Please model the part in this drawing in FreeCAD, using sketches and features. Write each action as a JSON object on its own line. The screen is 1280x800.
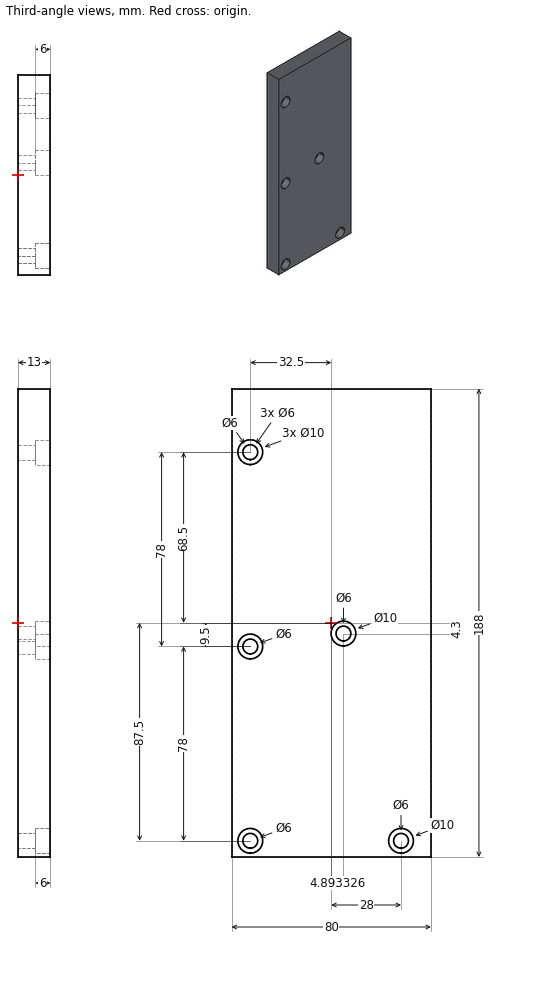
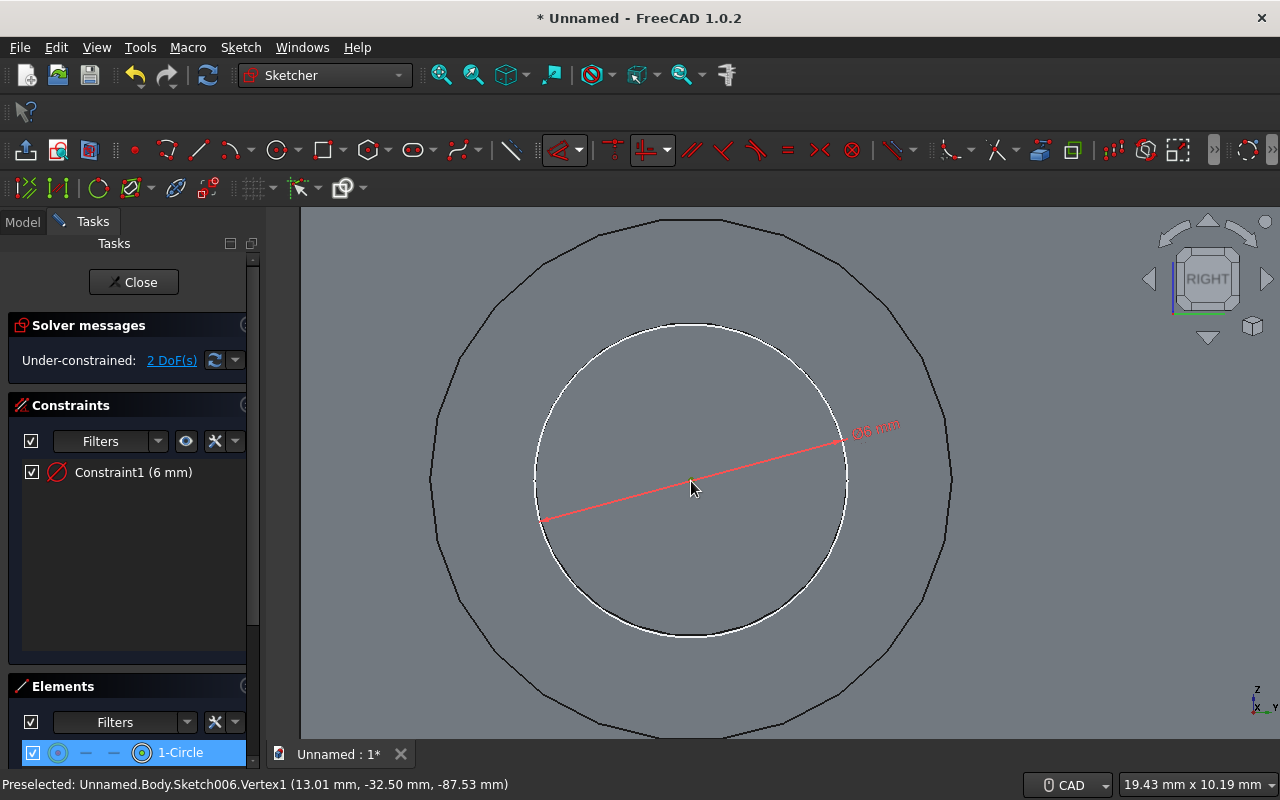
{"action": "left_click", "coordinate": [582, 150]}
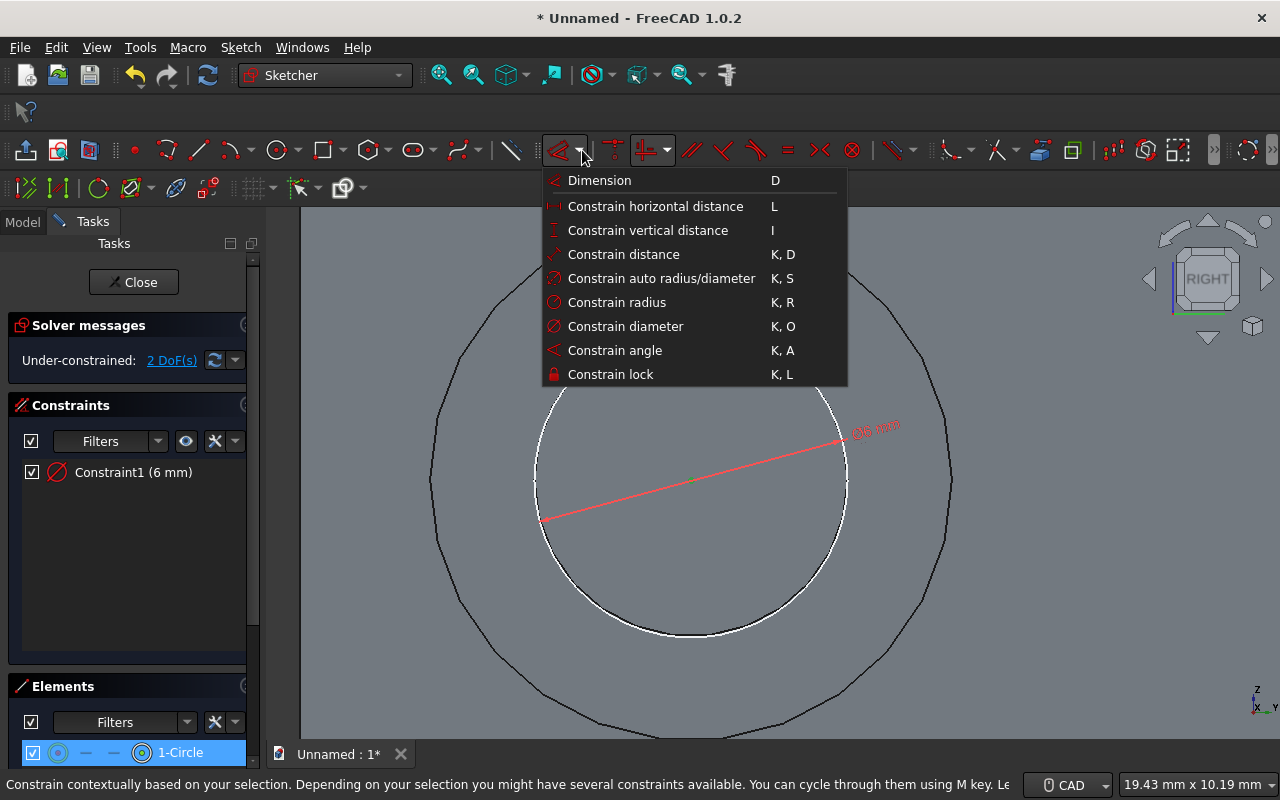
{"action": "left_click", "coordinate": [695, 206]}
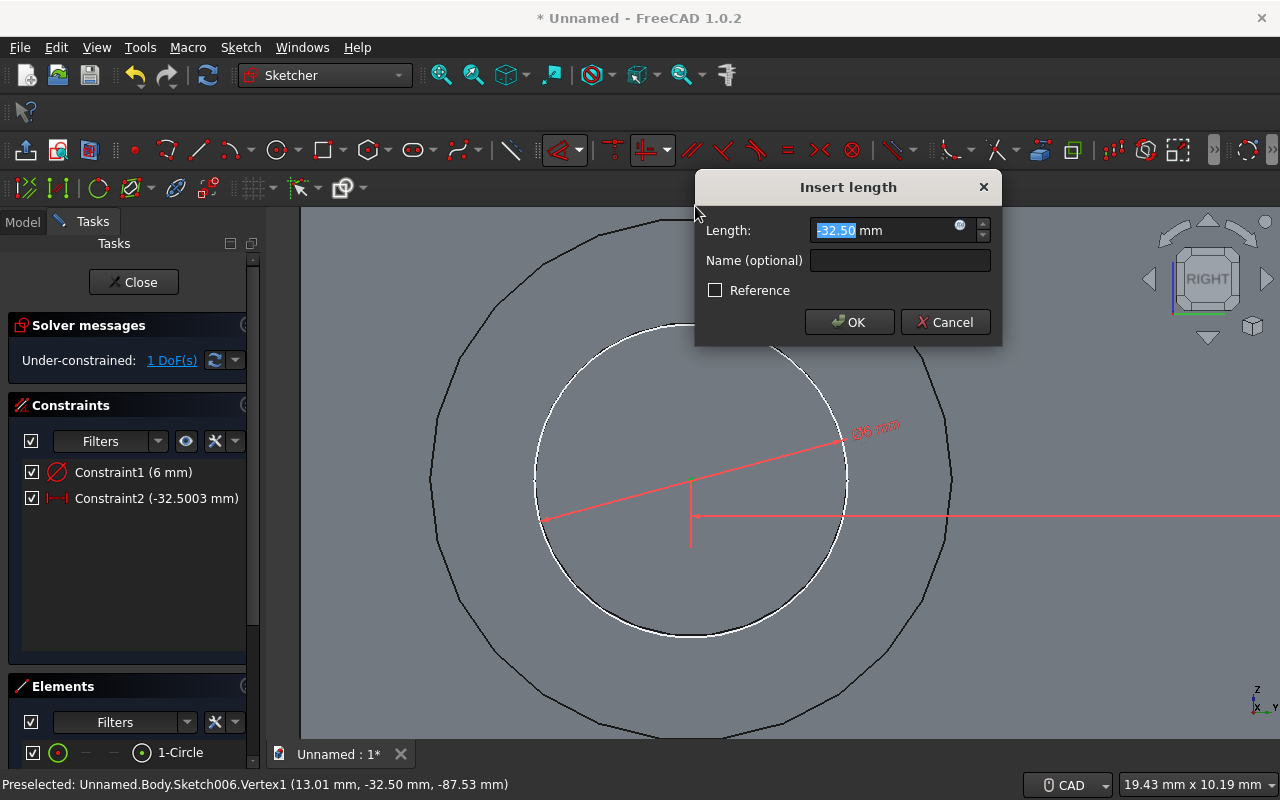
{"action": "type", "text": "-32.5"}
{"action": "key", "text": "Return"}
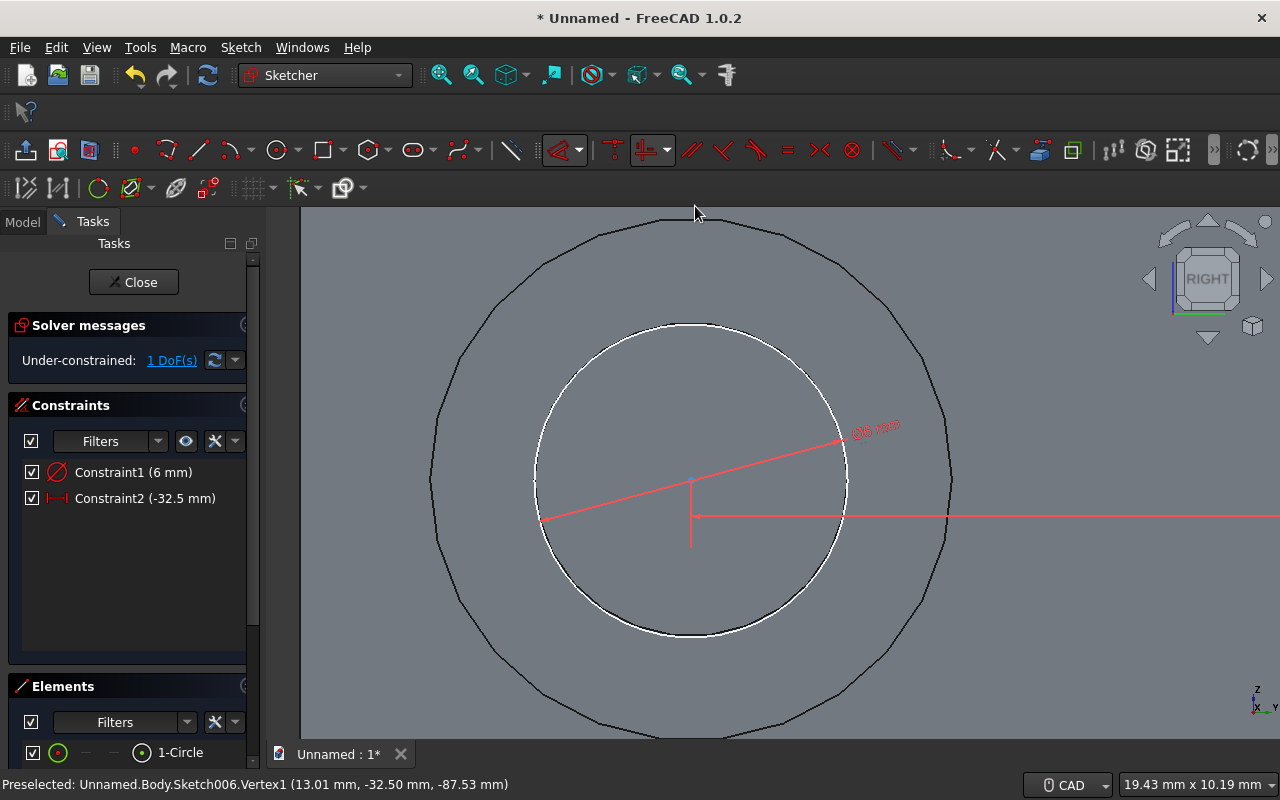
{"action": "left_click", "coordinate": [691, 481]}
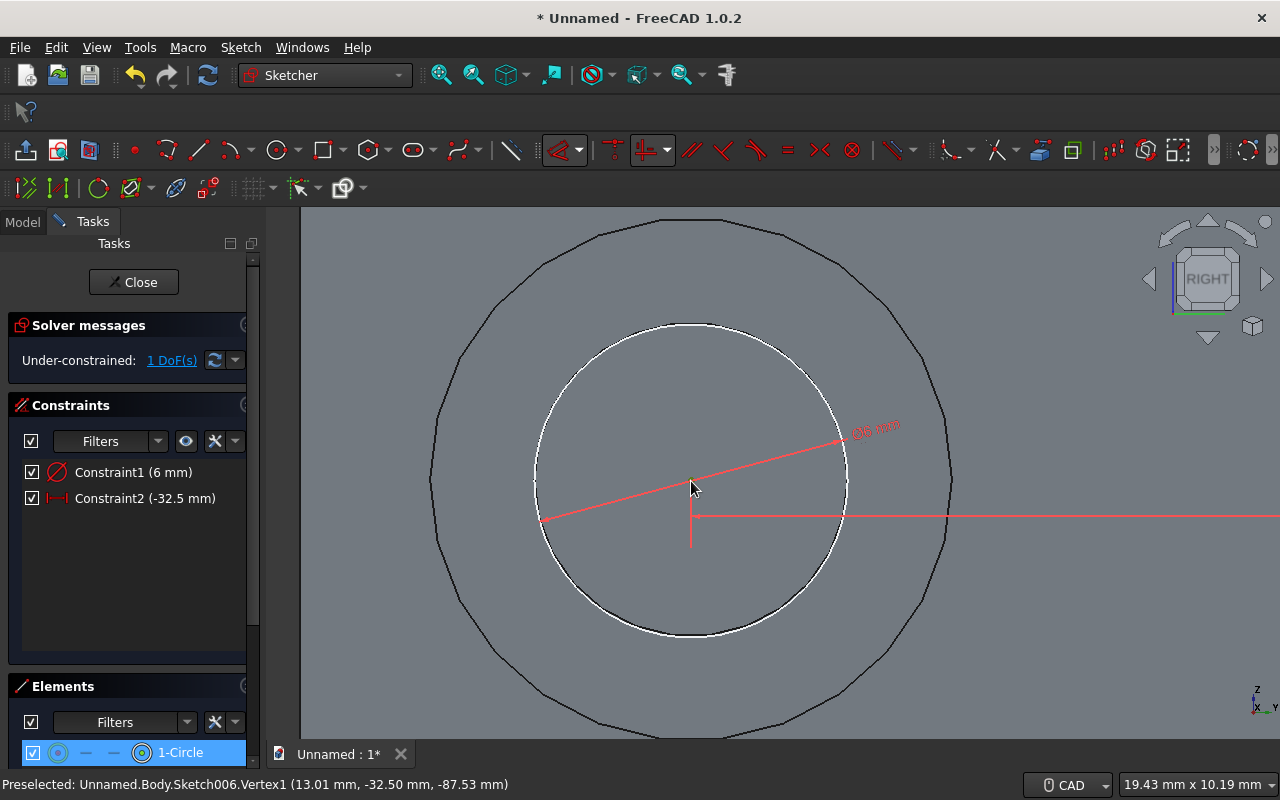
{"action": "left_click", "coordinate": [582, 150]}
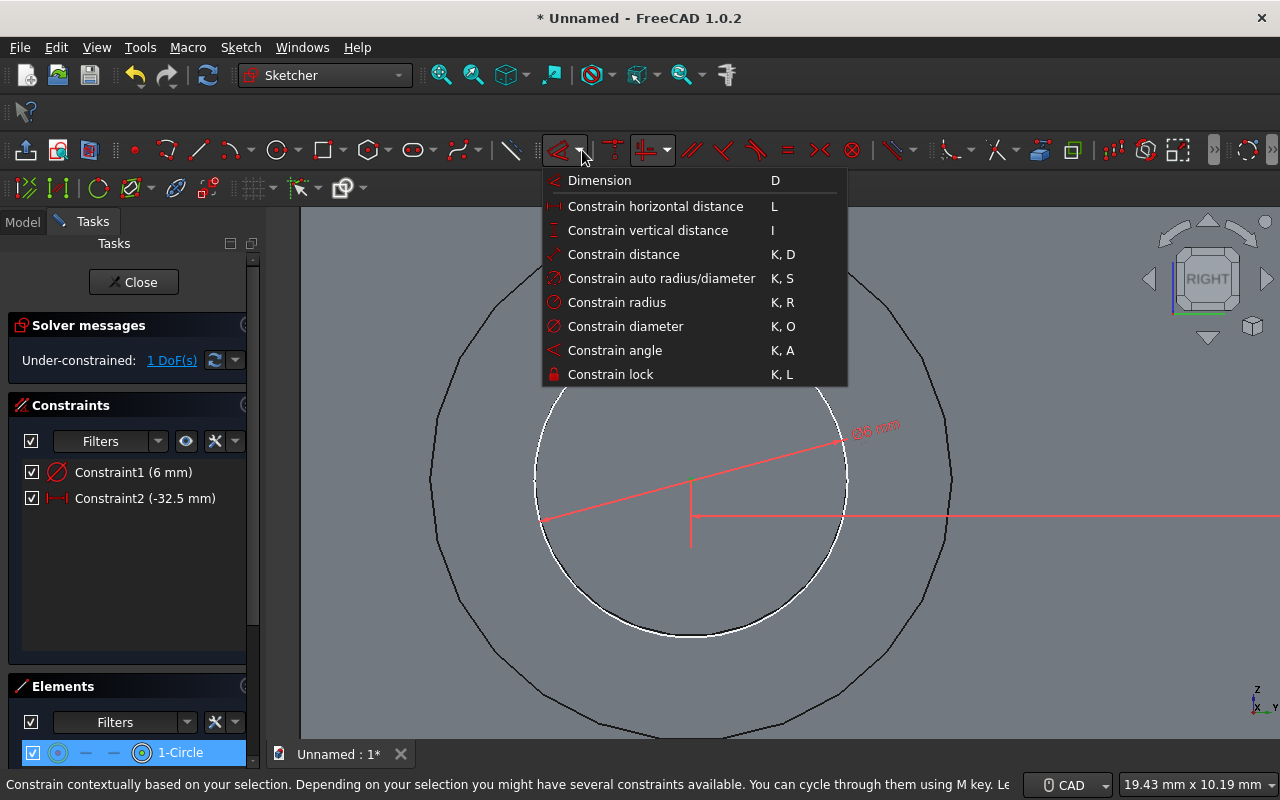
{"action": "left_click", "coordinate": [695, 230]}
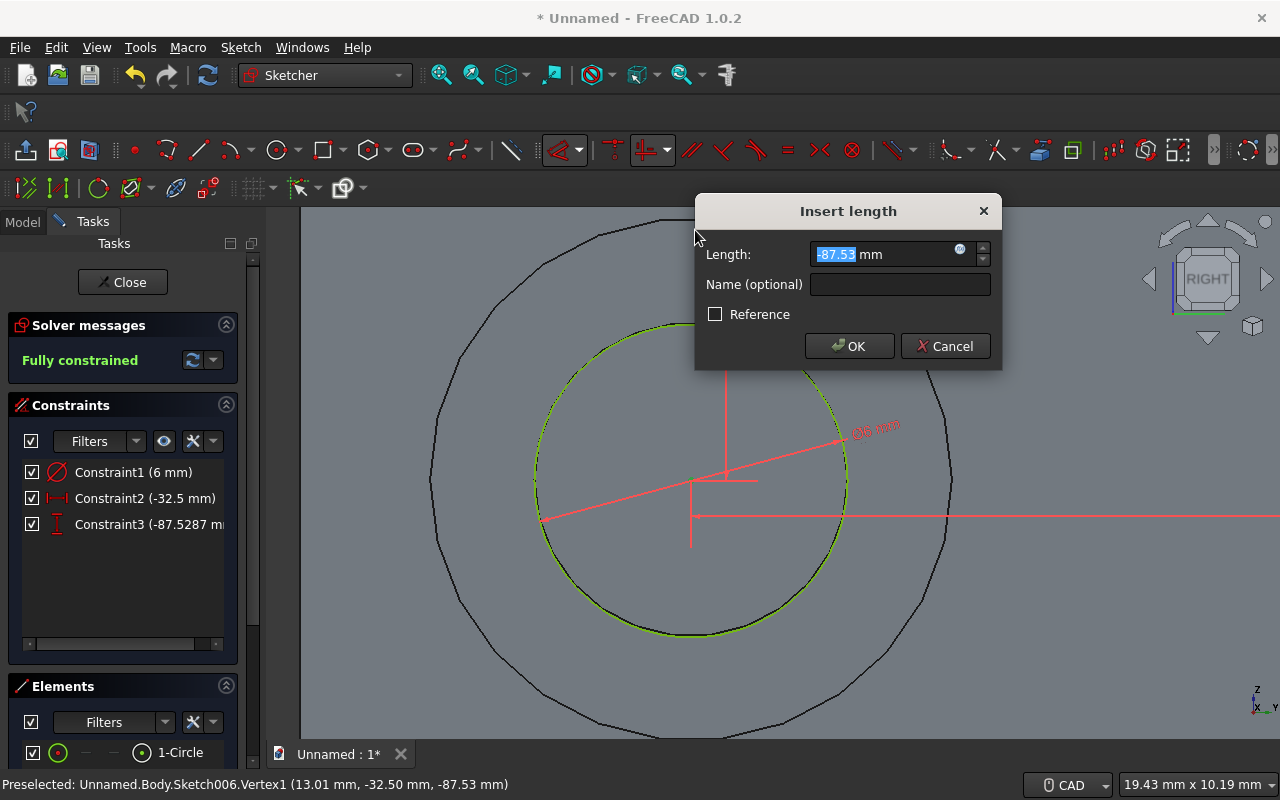
{"action": "type", "text": "-87.5"}
{"action": "key", "text": "Return"}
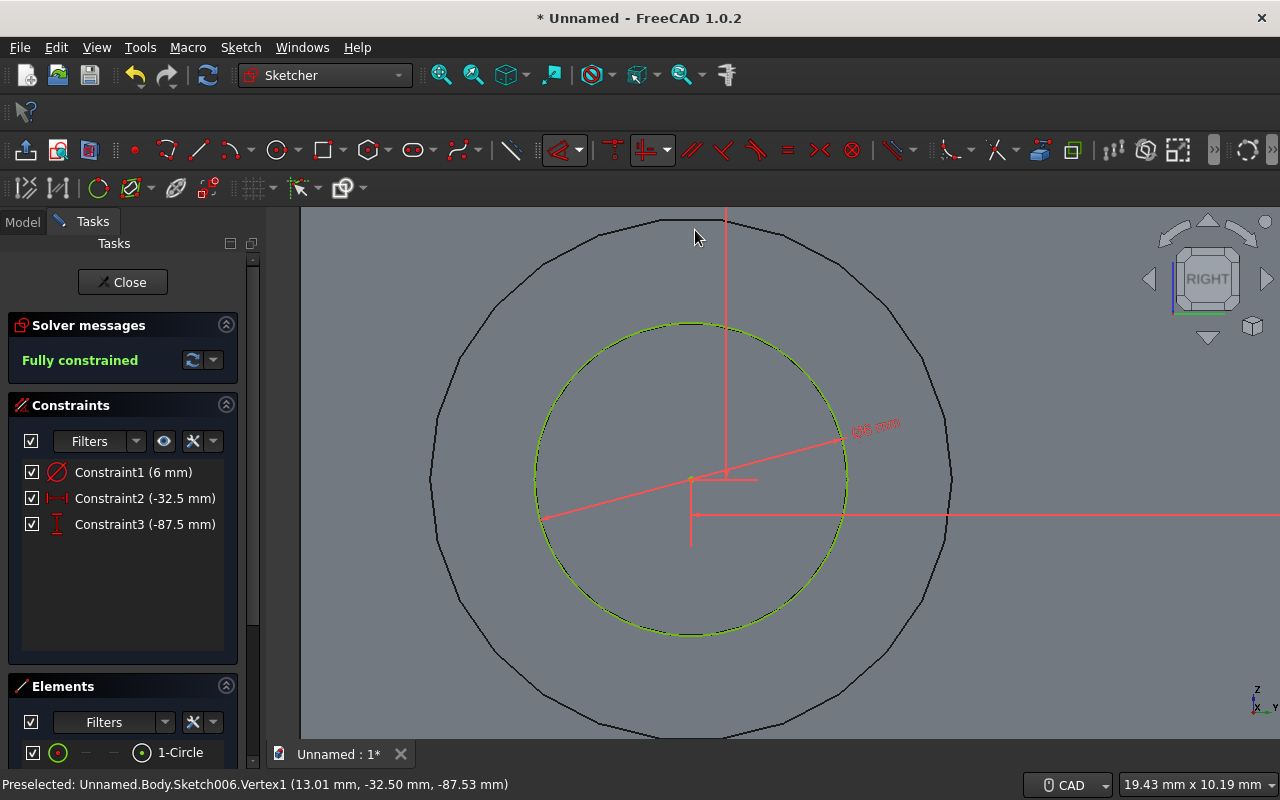
{"action": "left_click", "coordinate": [123, 282]}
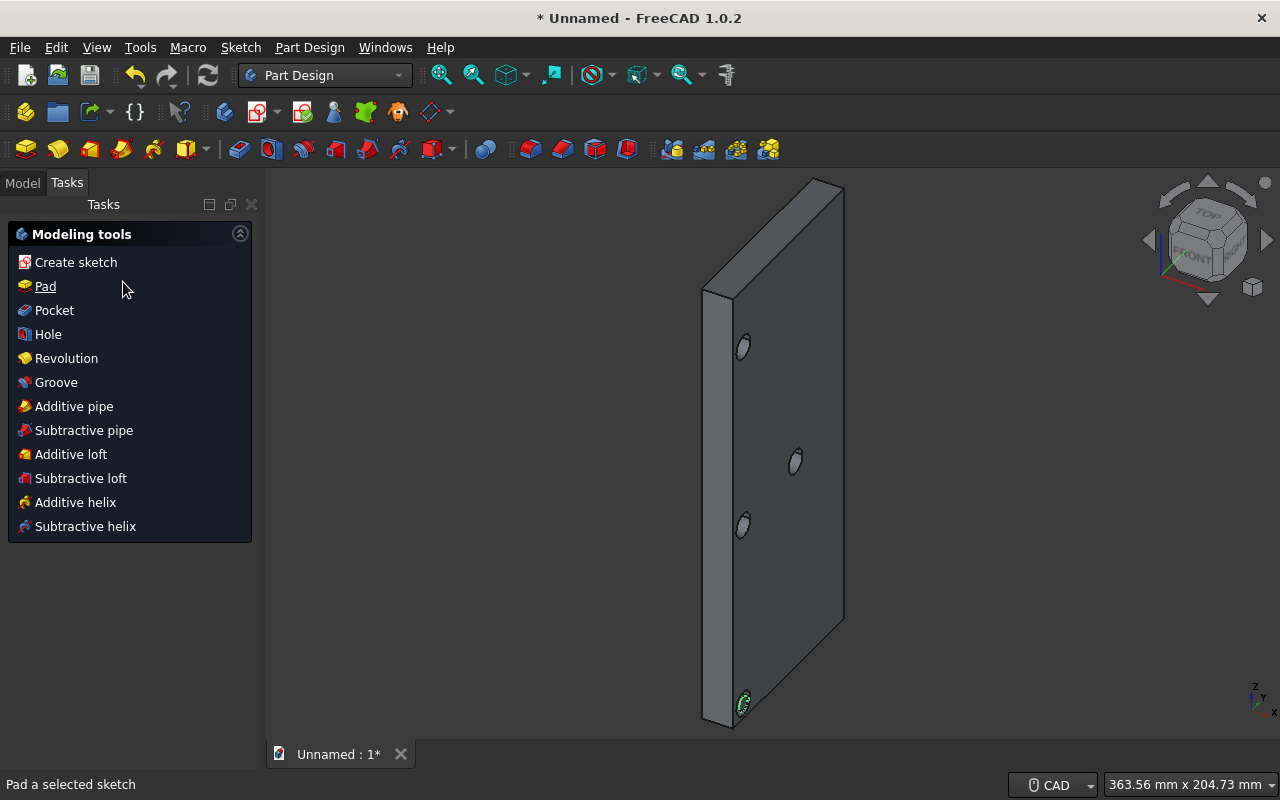
{"action": "left_click", "coordinate": [240, 150]}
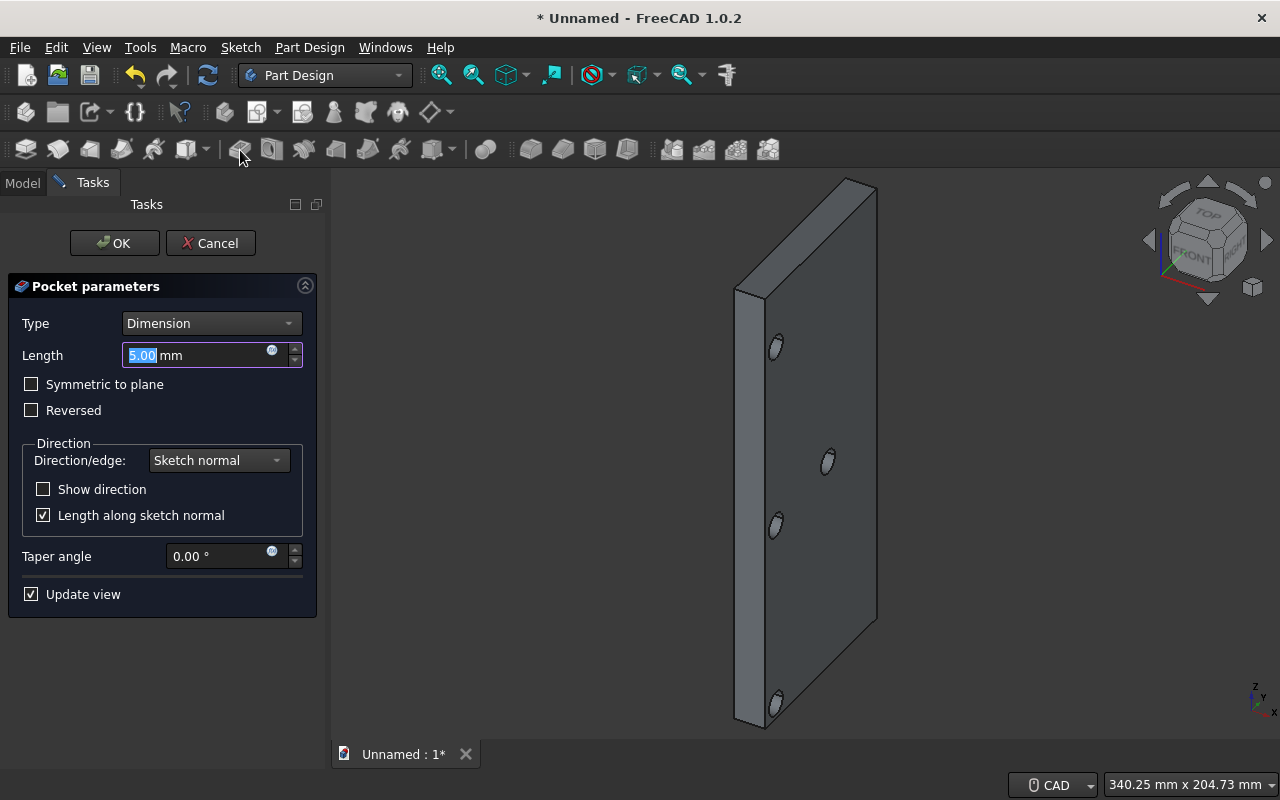
{"action": "left_click", "coordinate": [212, 324]}